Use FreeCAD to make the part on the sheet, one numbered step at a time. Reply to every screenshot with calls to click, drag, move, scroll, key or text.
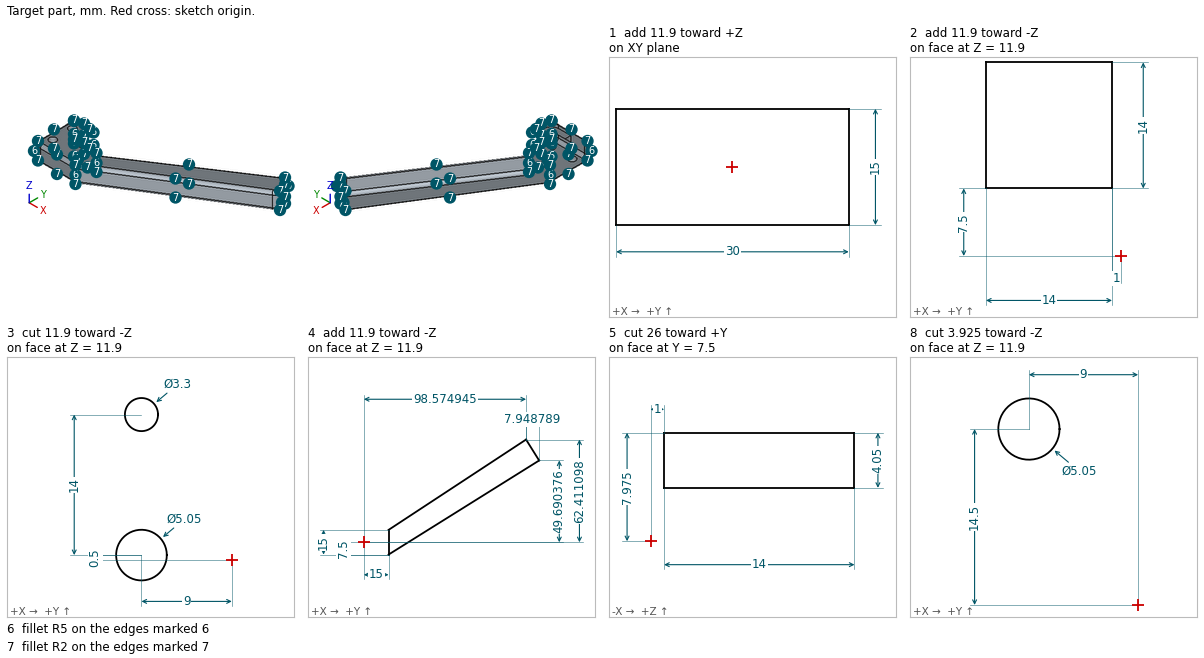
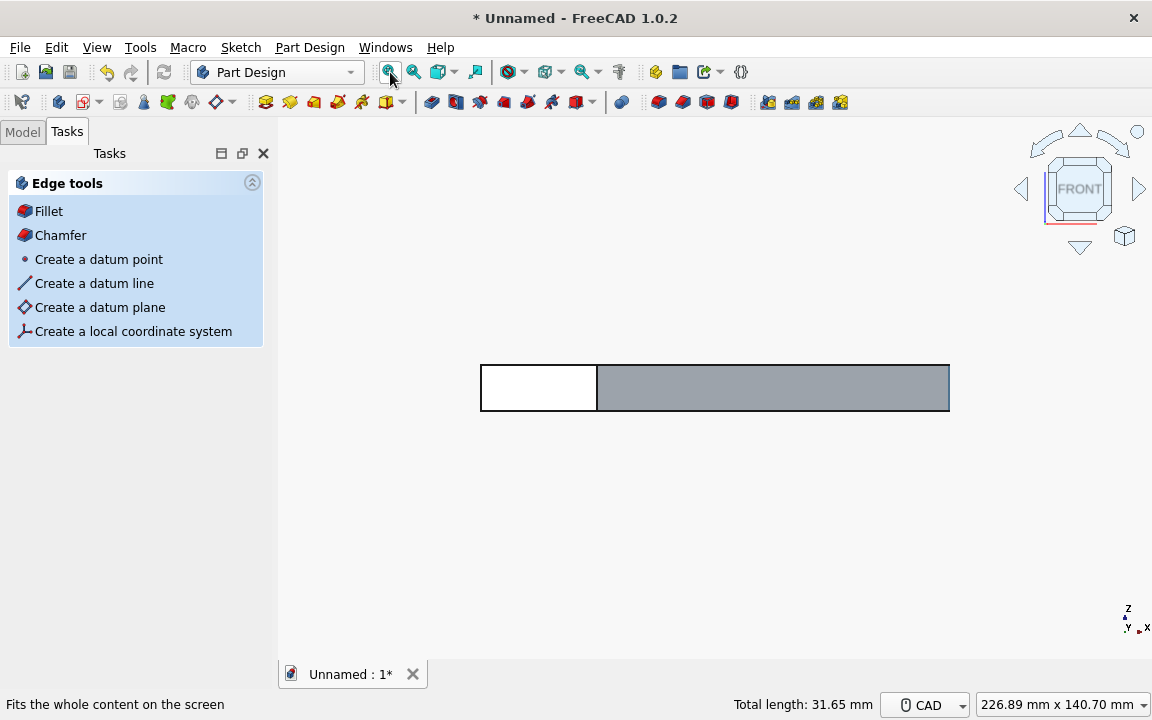
click(597, 387, ctrl)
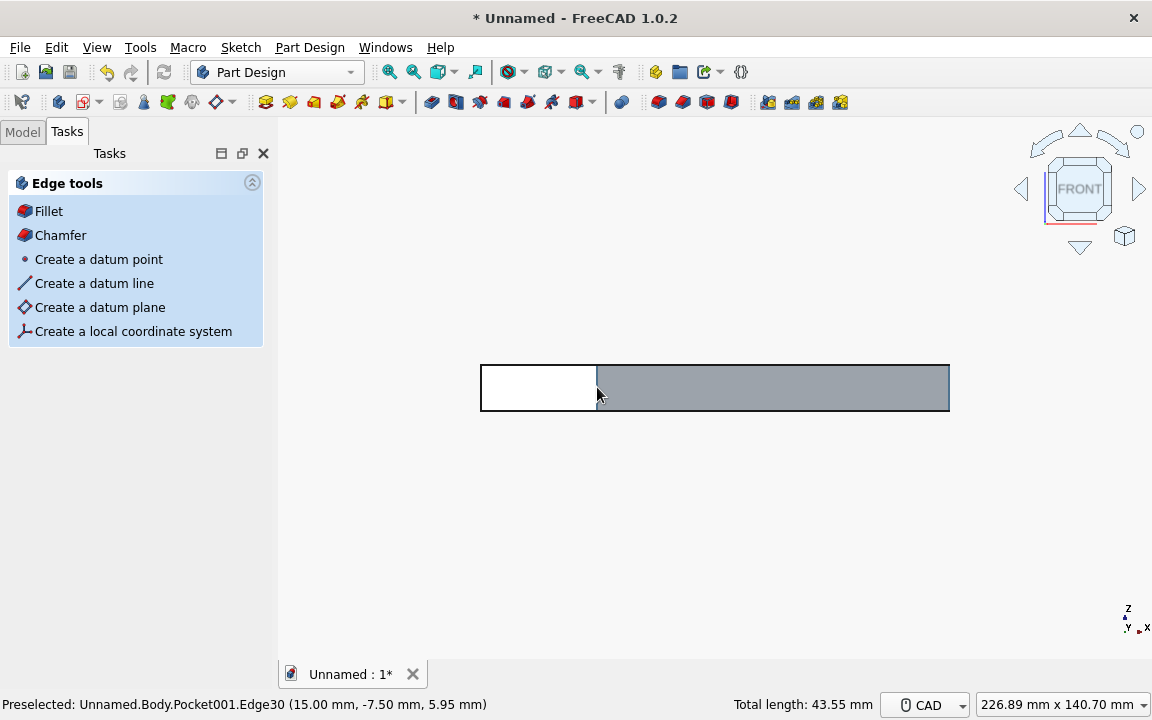
click(481, 387, ctrl)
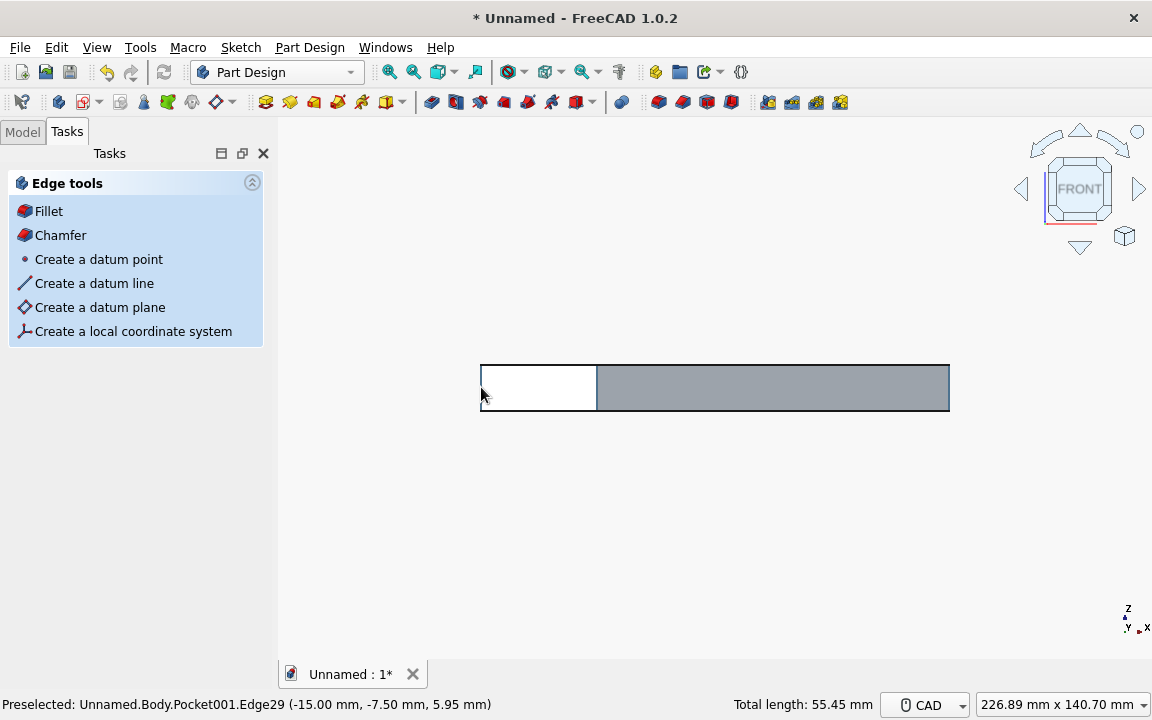
scroll(535, 402, up, 5)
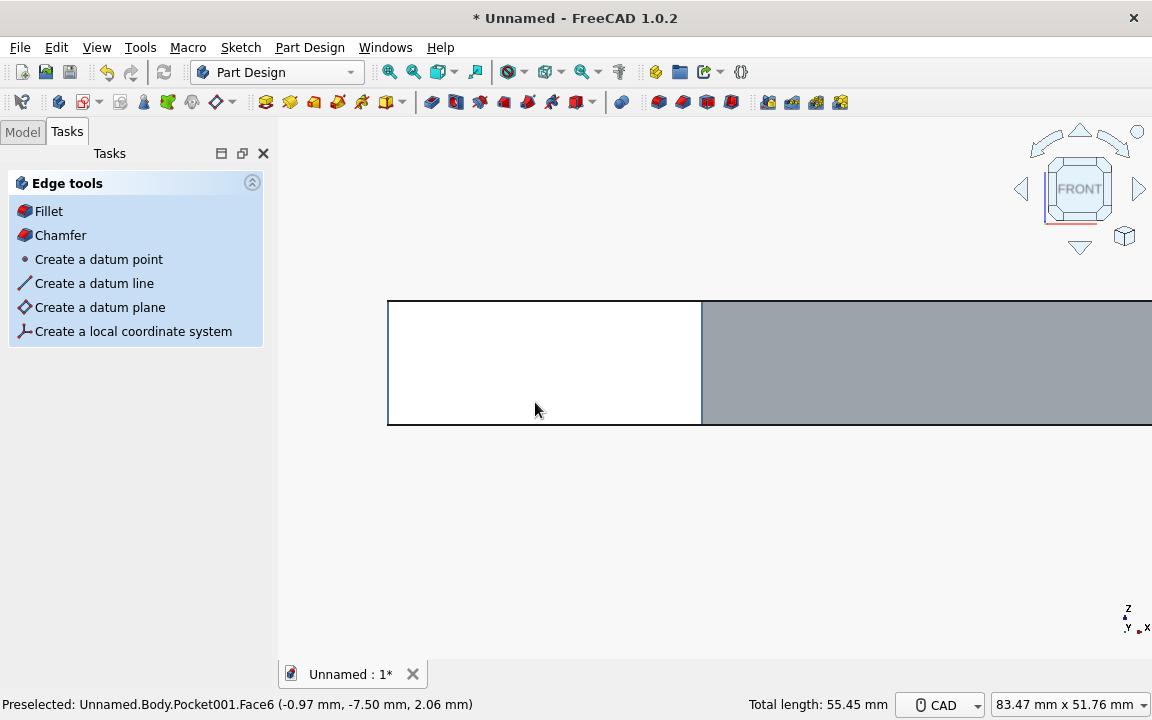
click(390, 72)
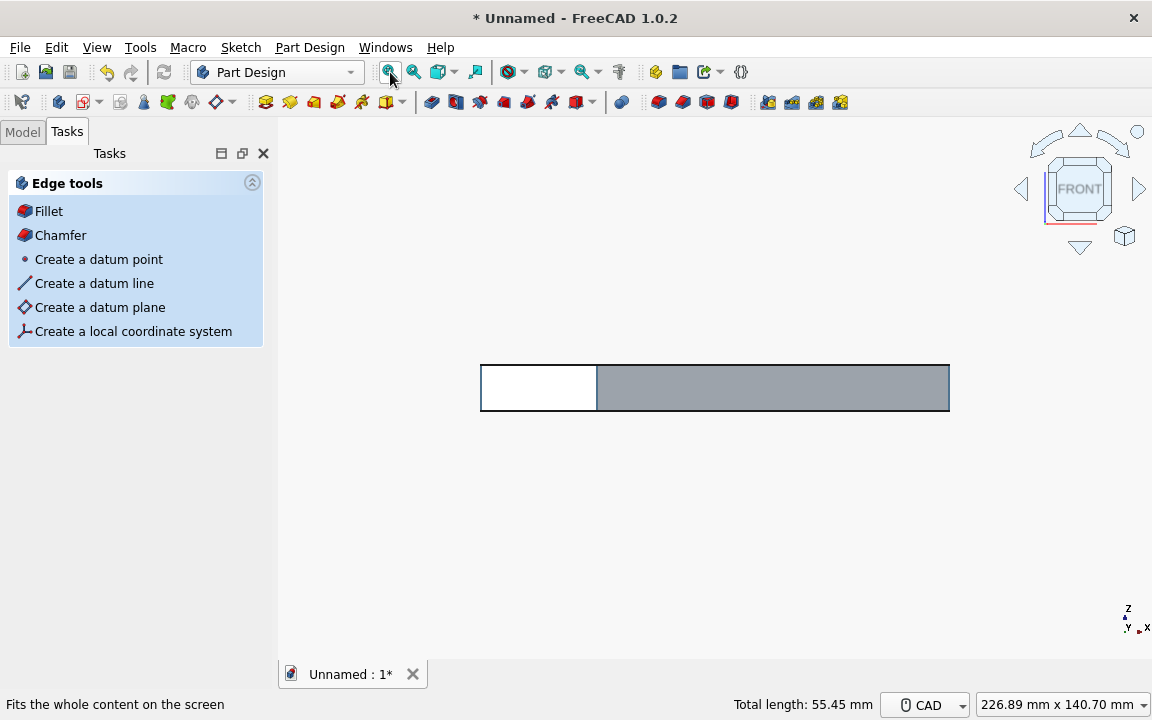
key(3)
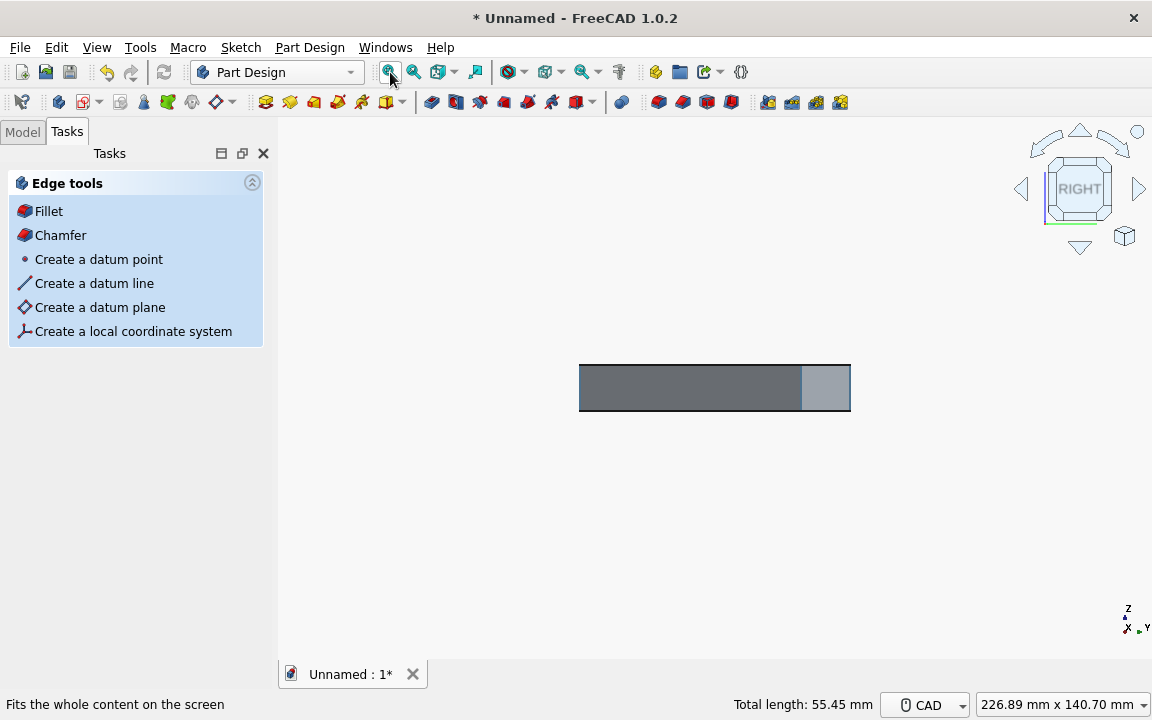
click(390, 72)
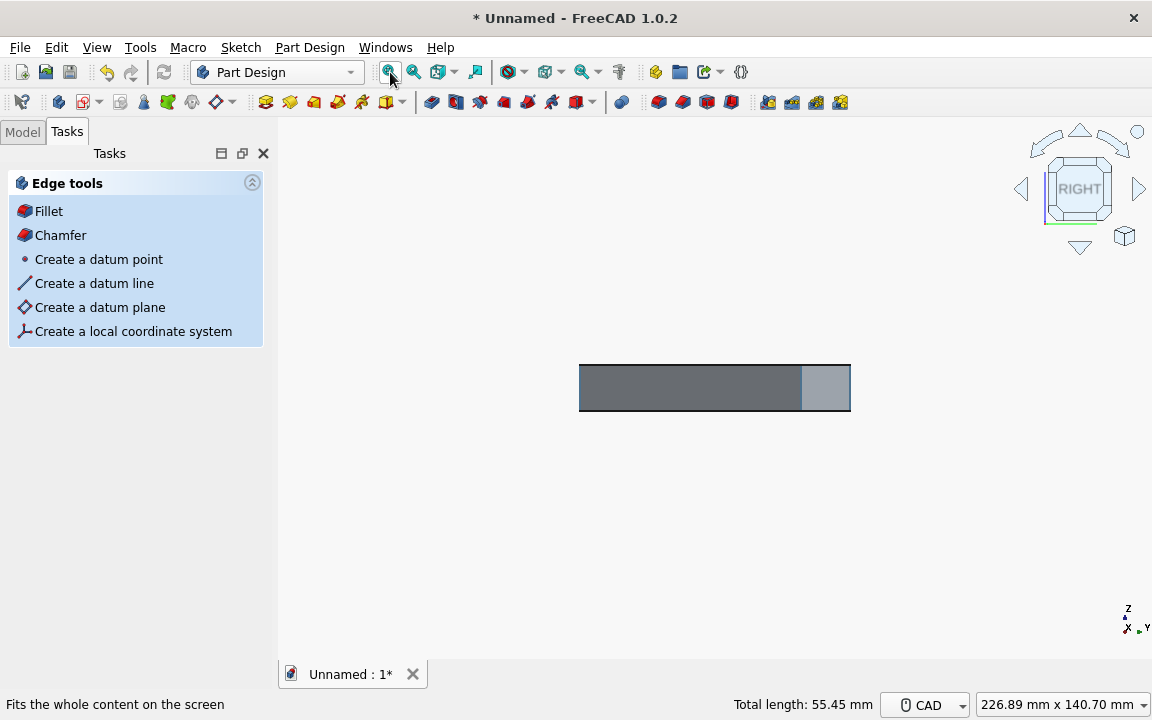
scroll(692, 402, up, 5)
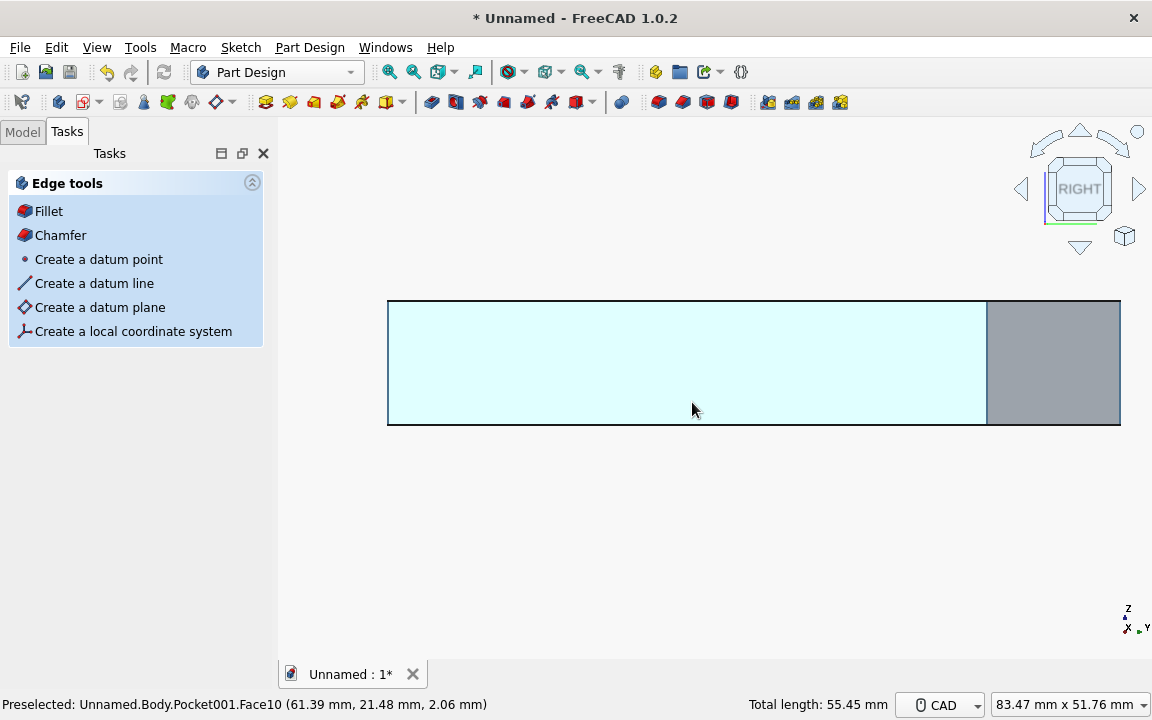
key(v)
key(f)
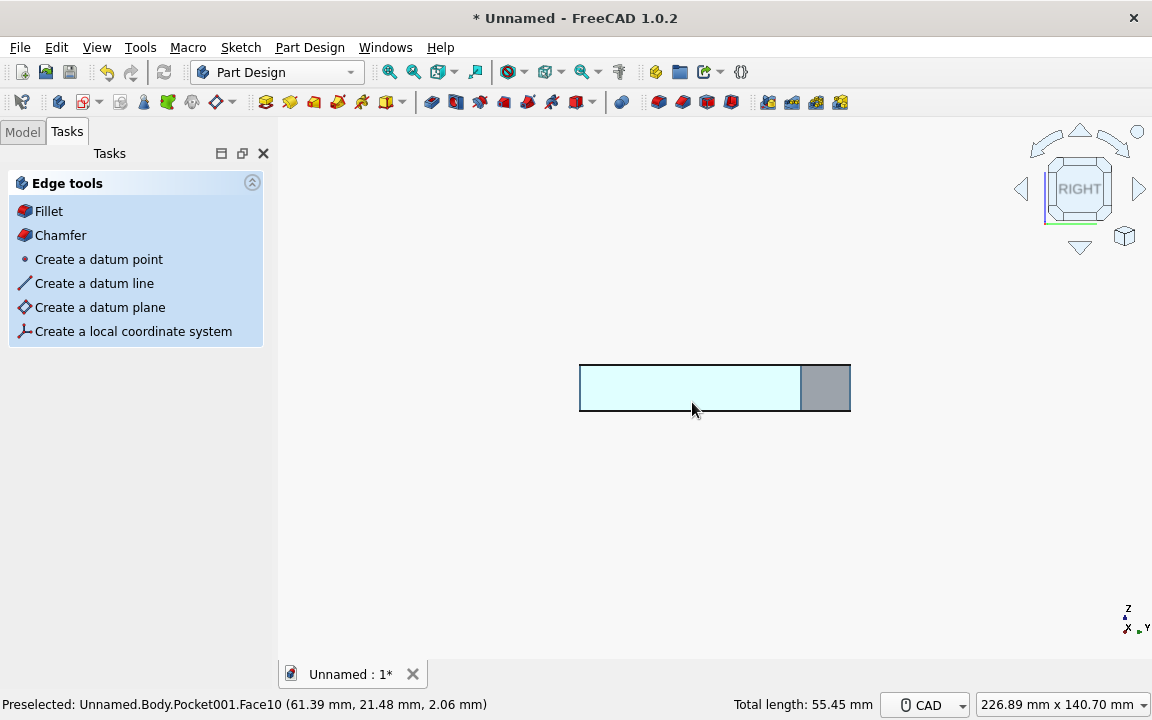
key(5)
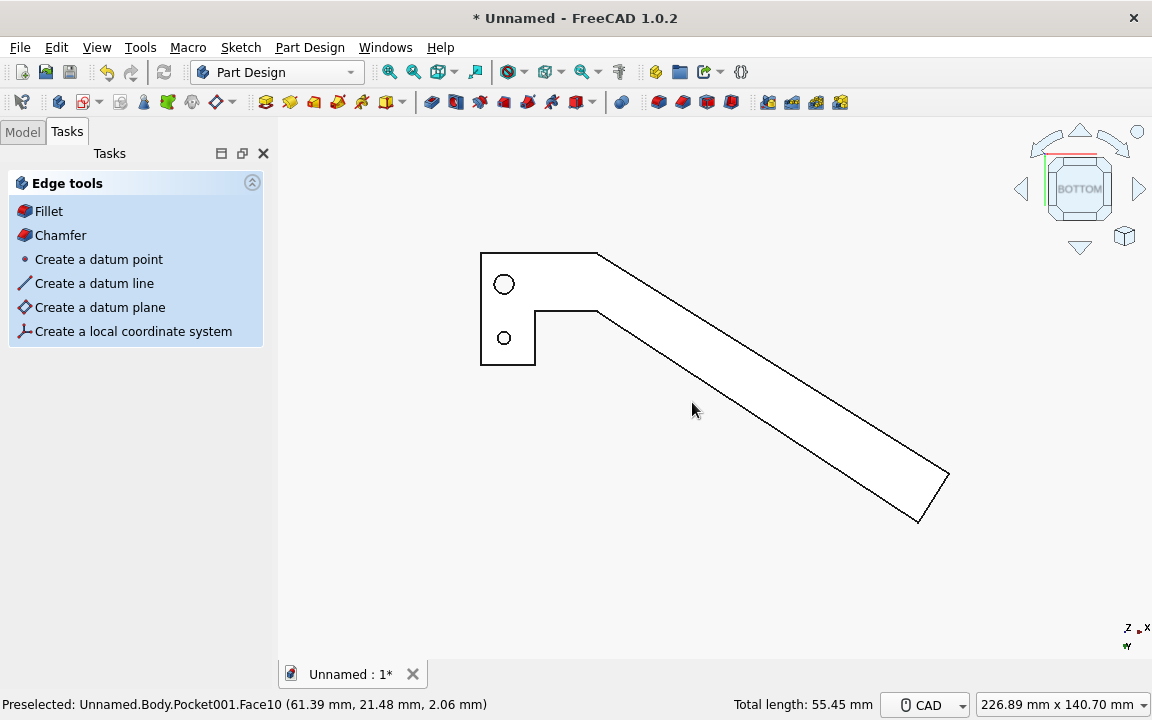
scroll(535, 364, up, 5)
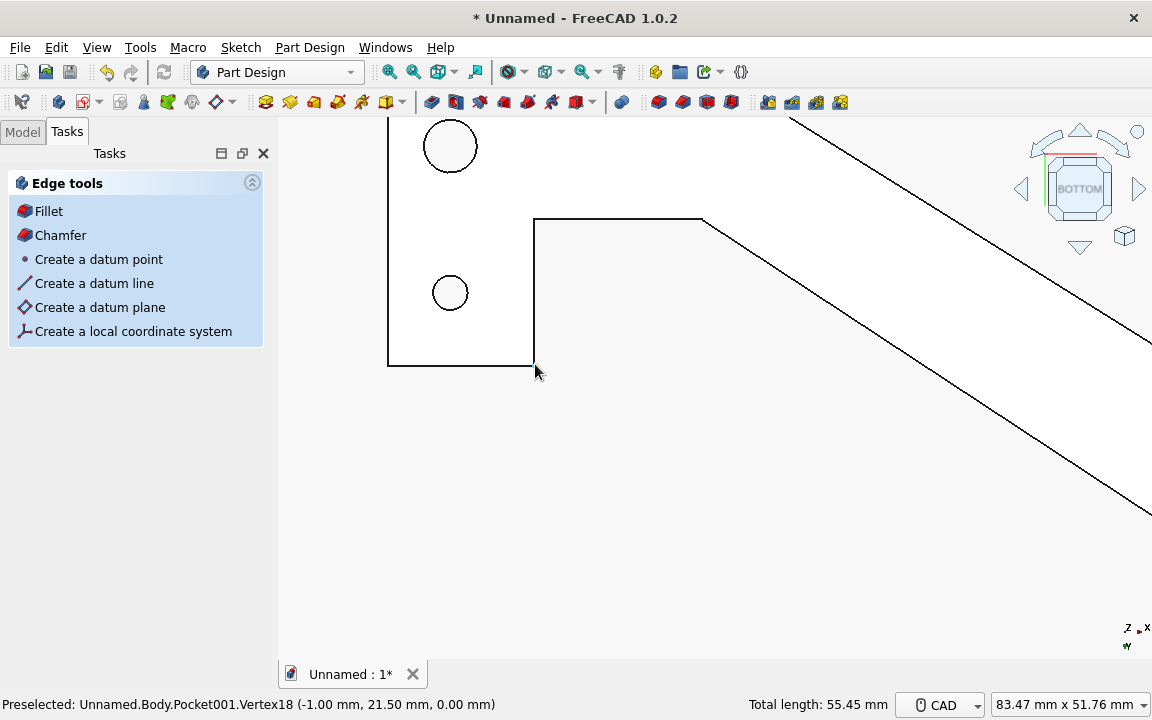
key(v)
key(f)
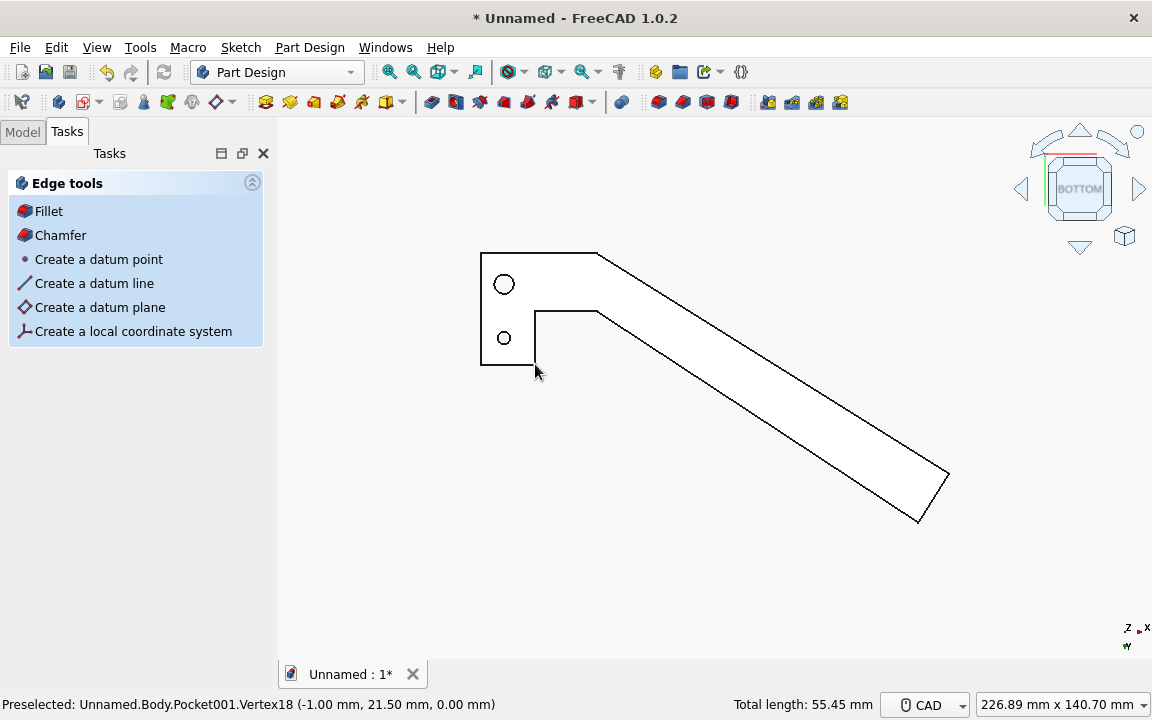
key(4)